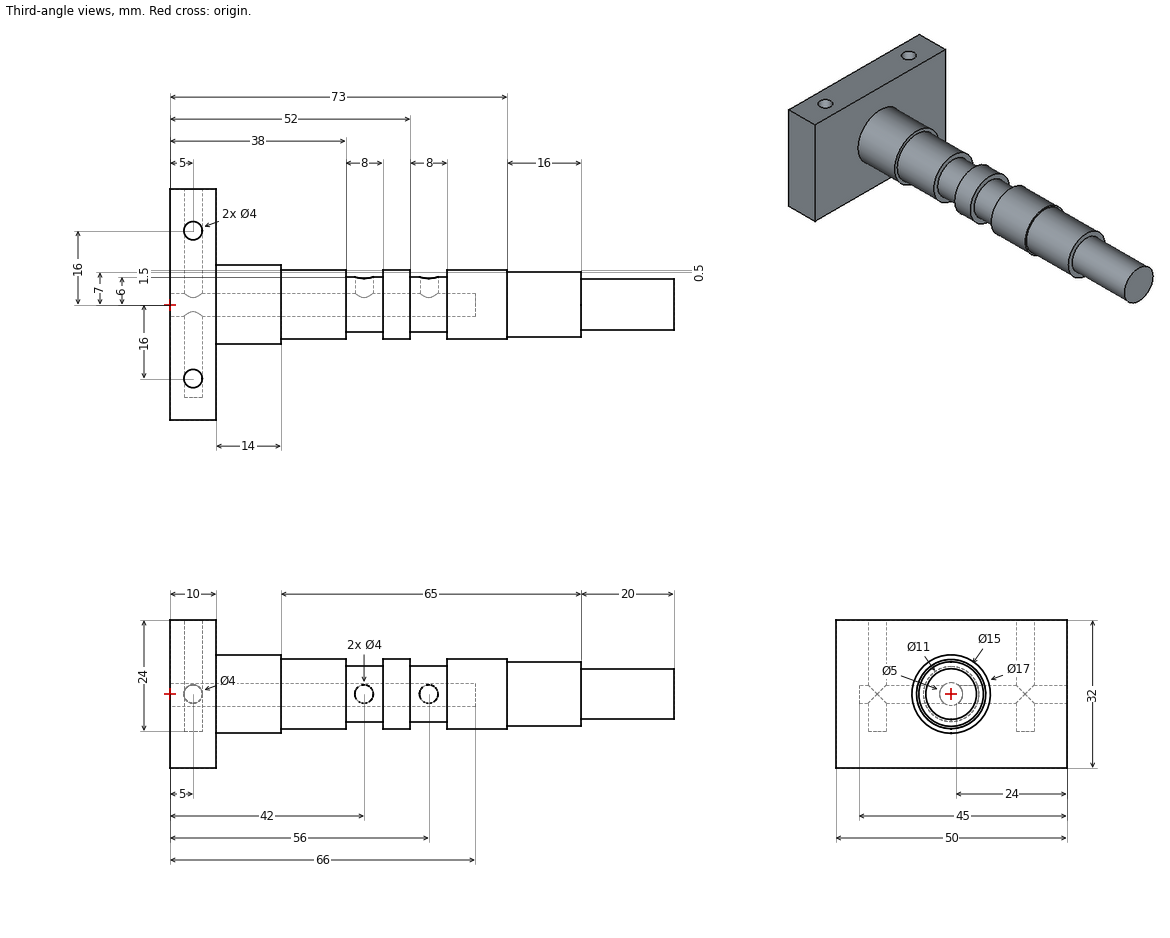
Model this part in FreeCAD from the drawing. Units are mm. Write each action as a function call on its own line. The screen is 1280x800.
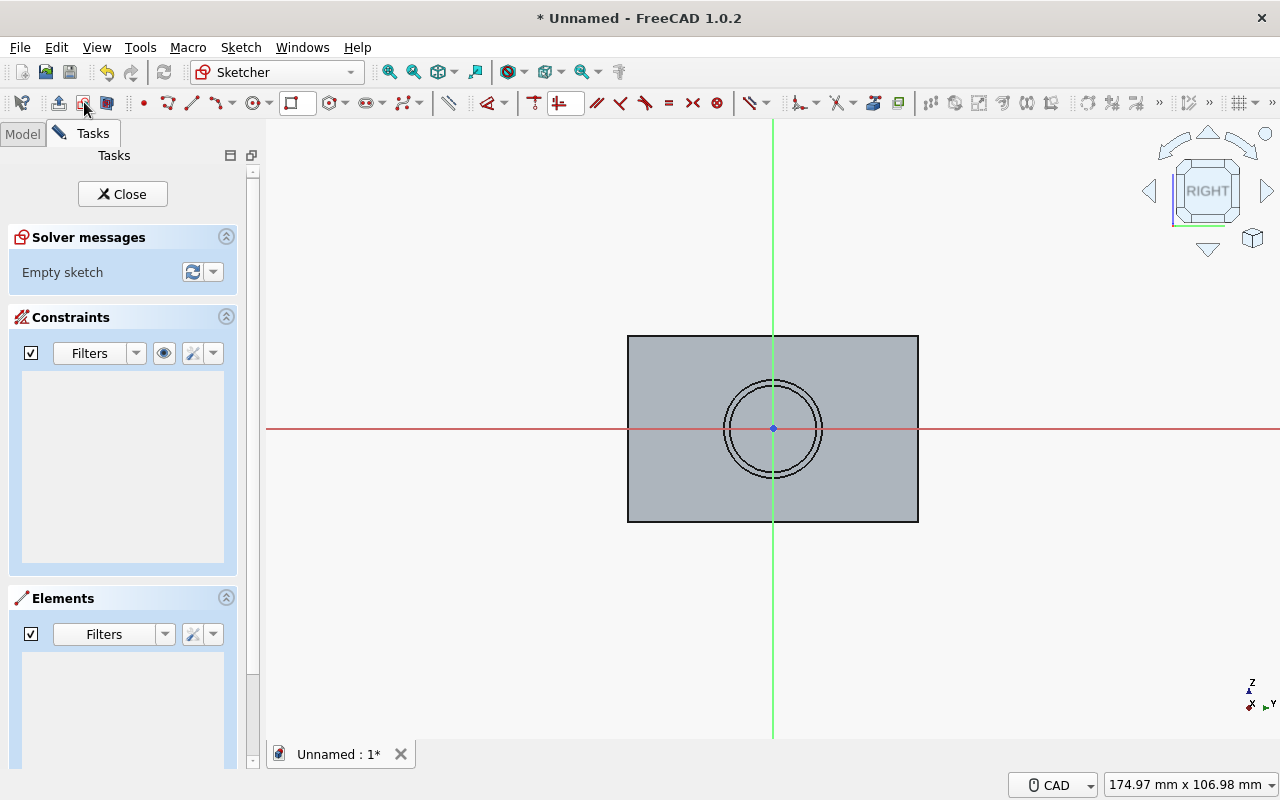
scroll(787, 429, up, 9)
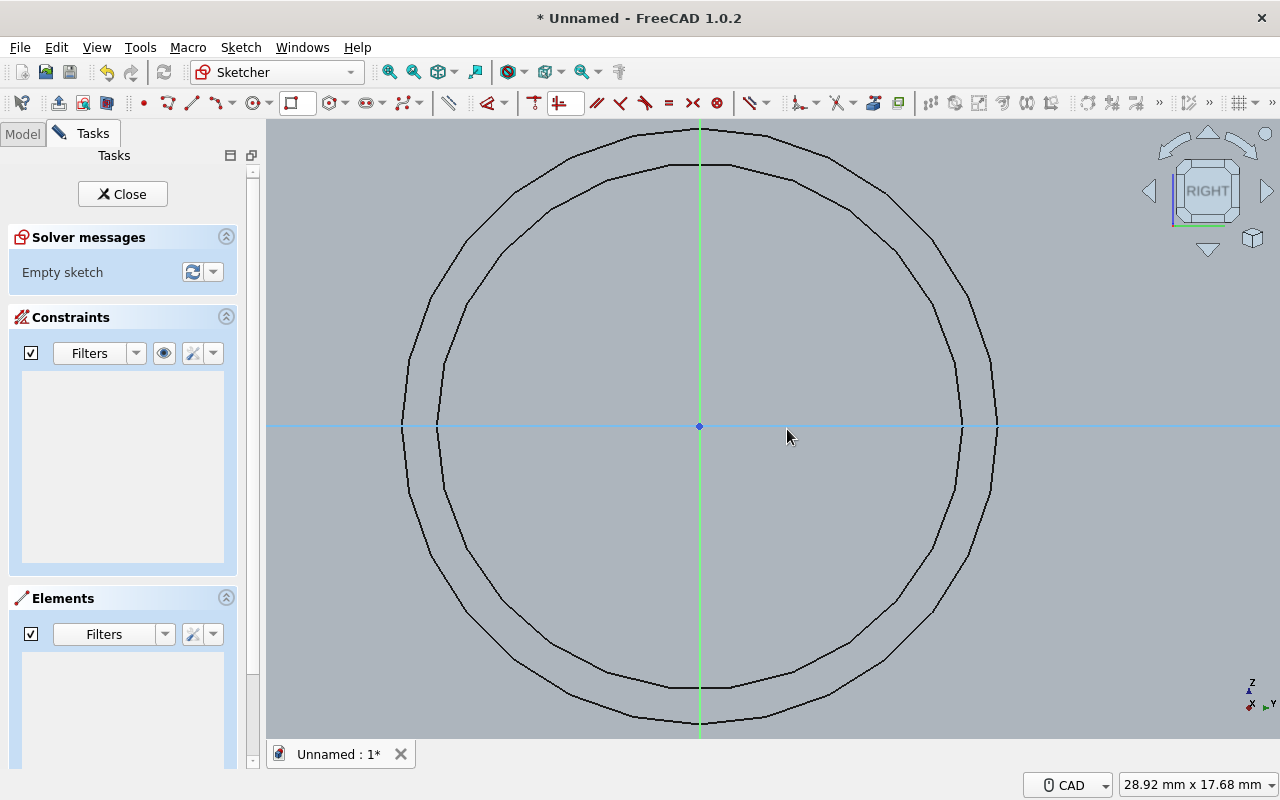
click(254, 104)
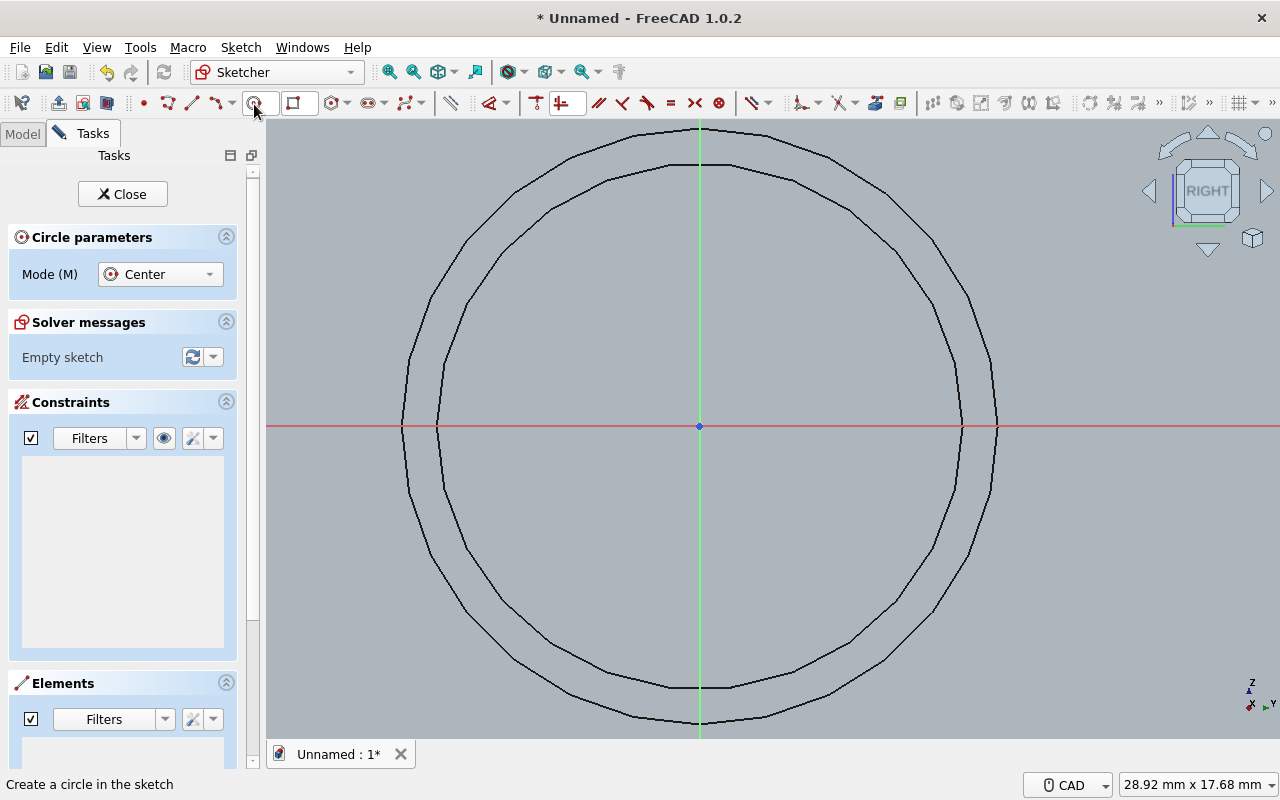
click(700, 426)
move(836, 290)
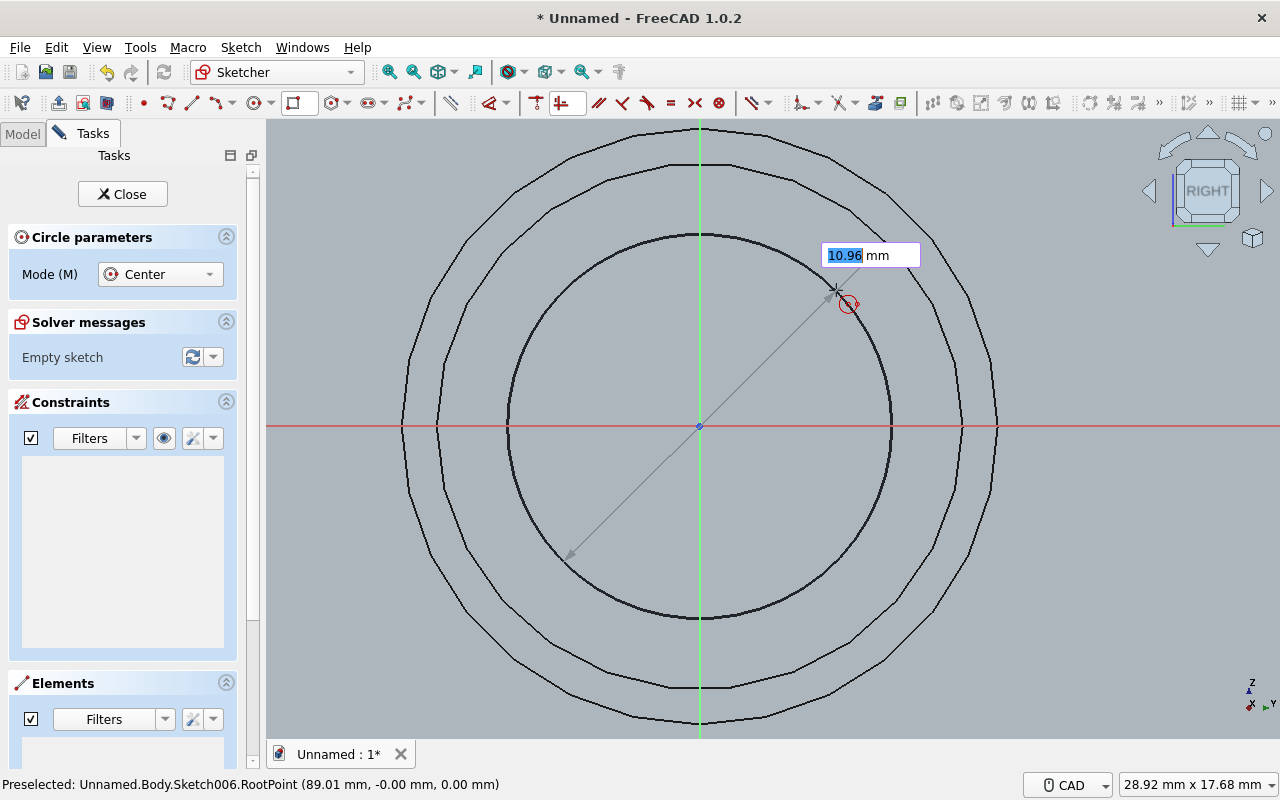
text(11)
key(Return)
key(Escape)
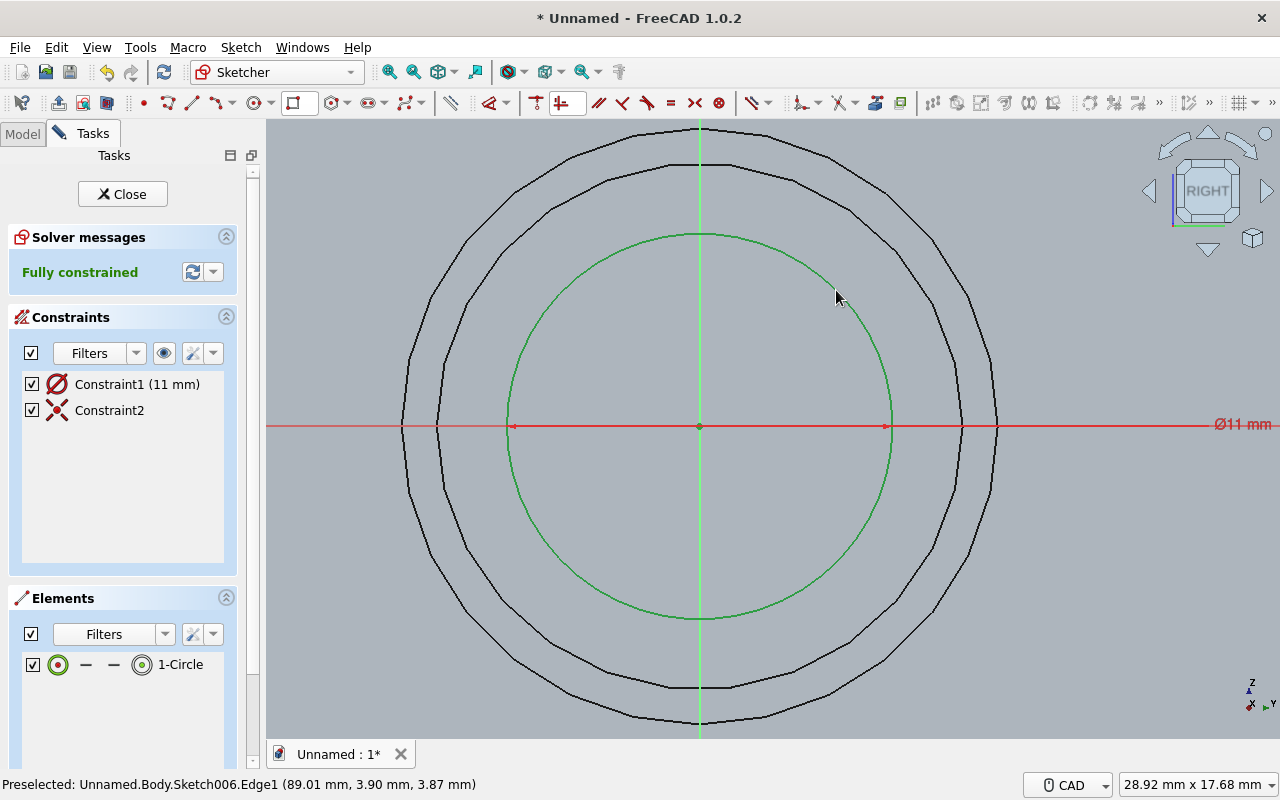
click(123, 194)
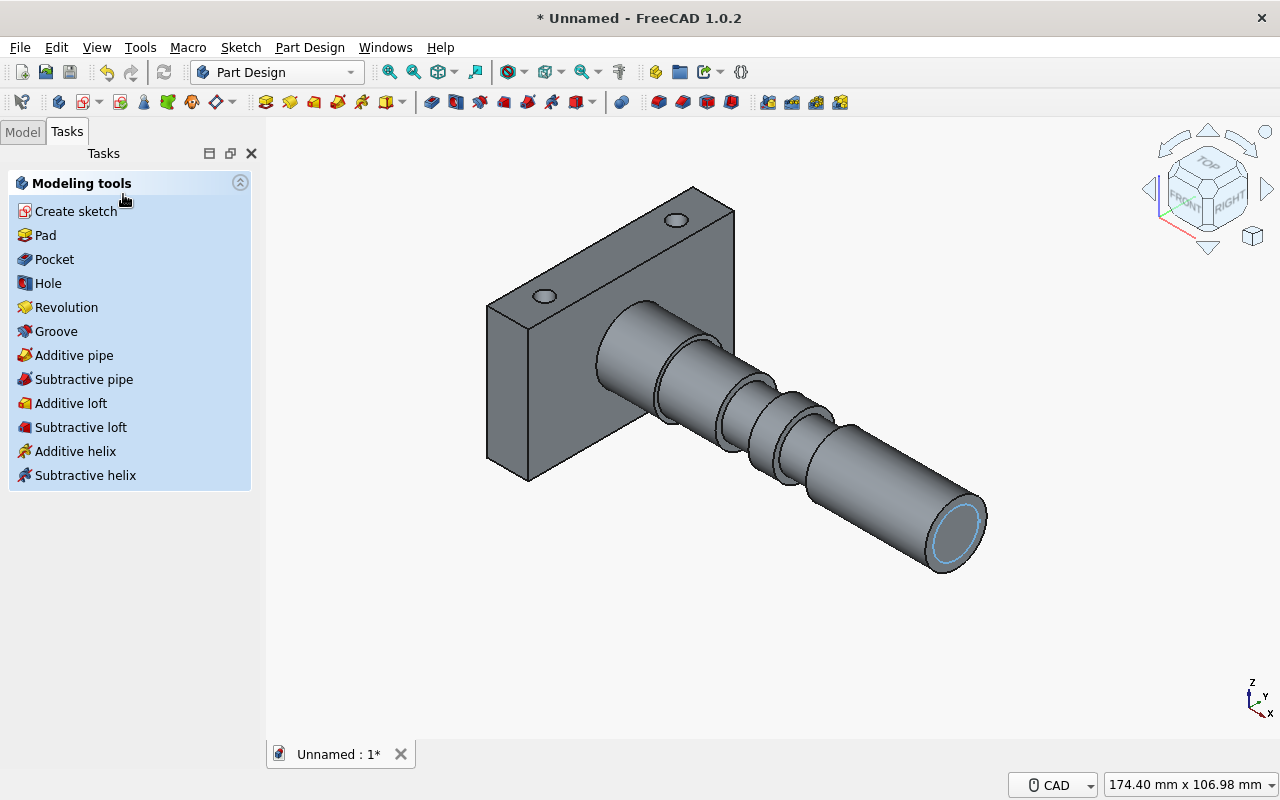
click(266, 102)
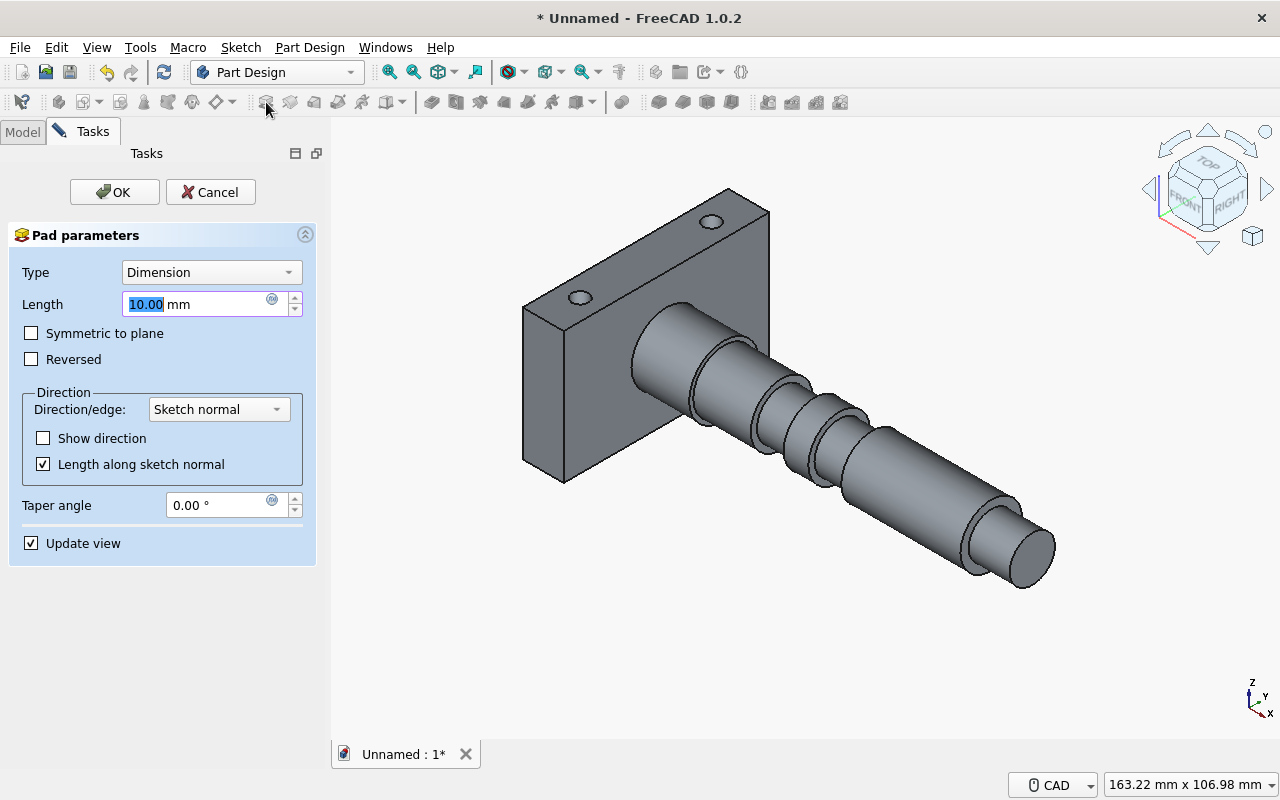
text(20)
key(Tab)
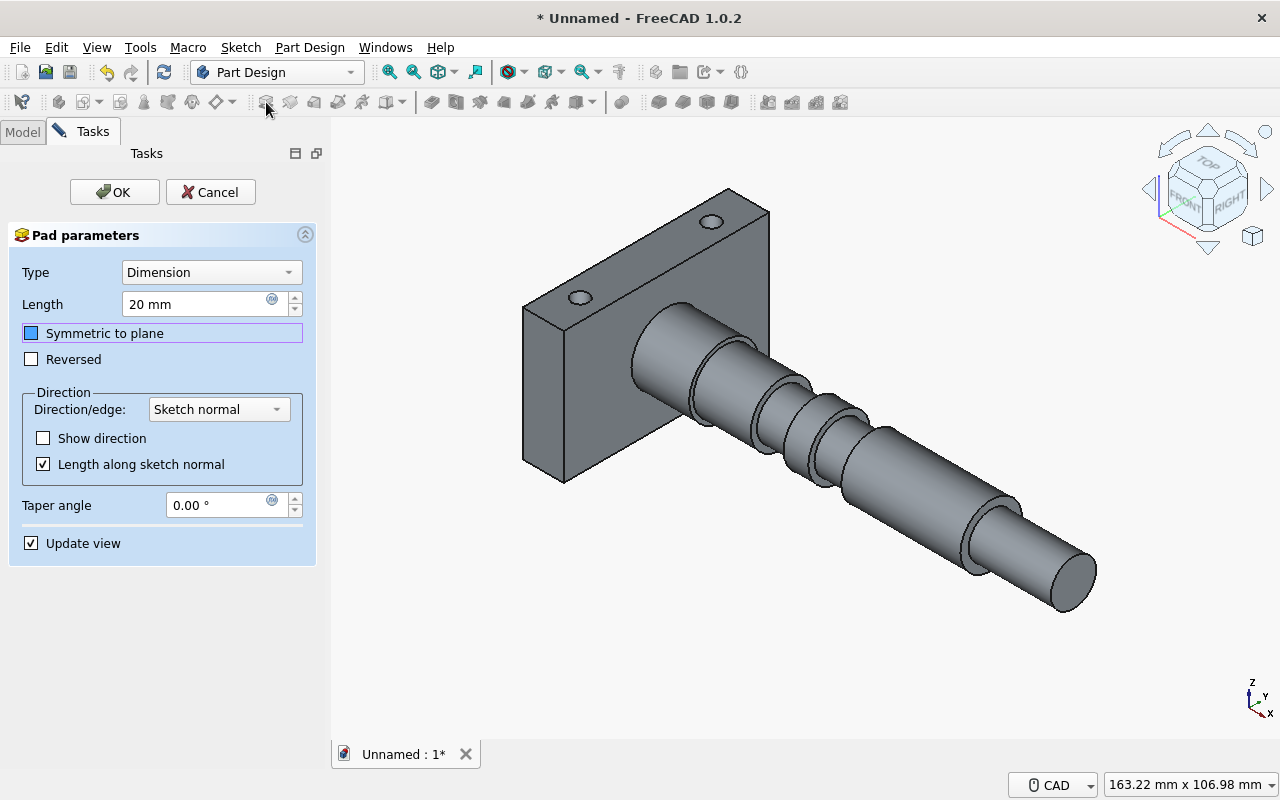
click(115, 192)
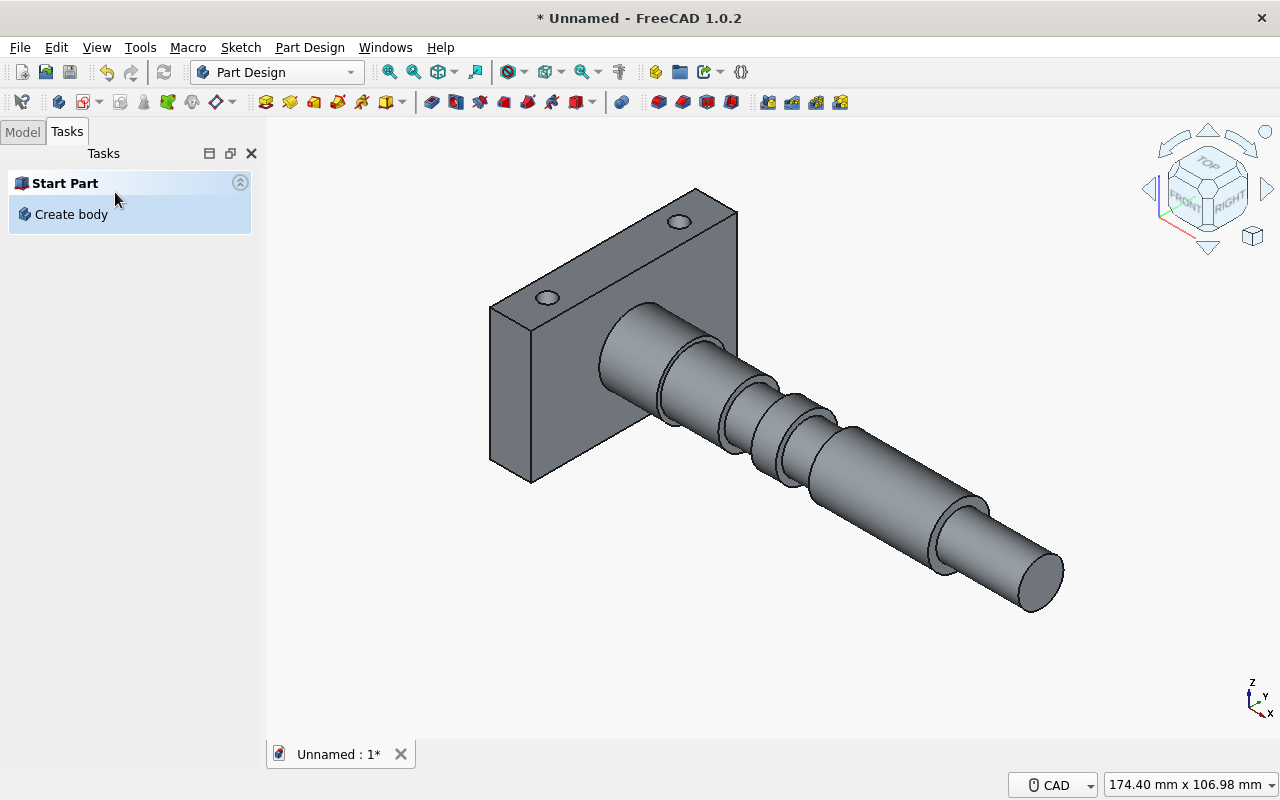
click(84, 102)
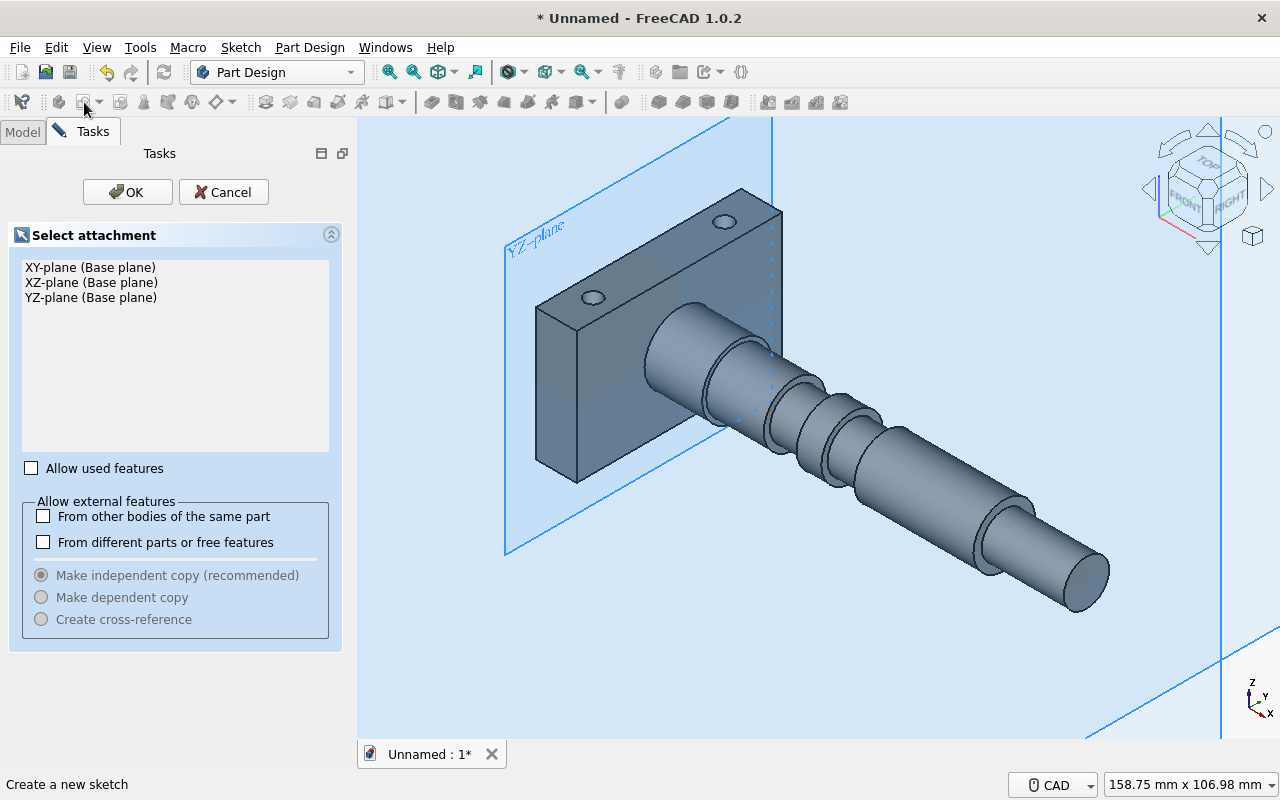
click(82, 268)